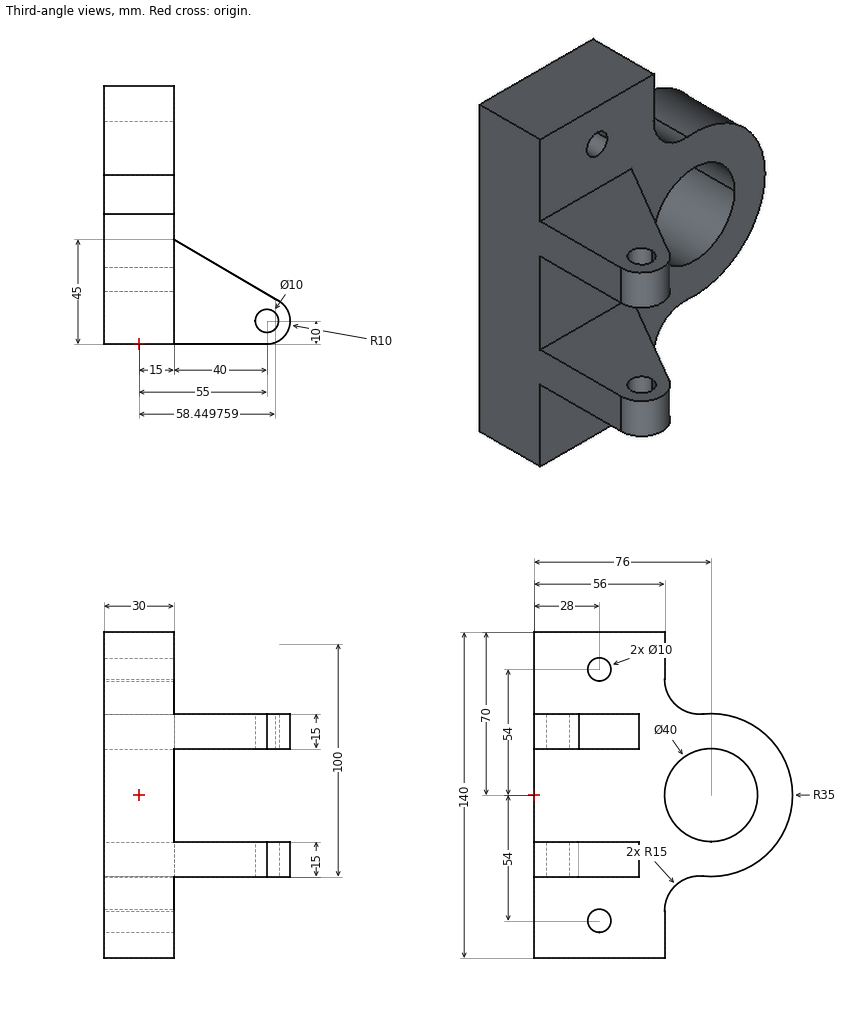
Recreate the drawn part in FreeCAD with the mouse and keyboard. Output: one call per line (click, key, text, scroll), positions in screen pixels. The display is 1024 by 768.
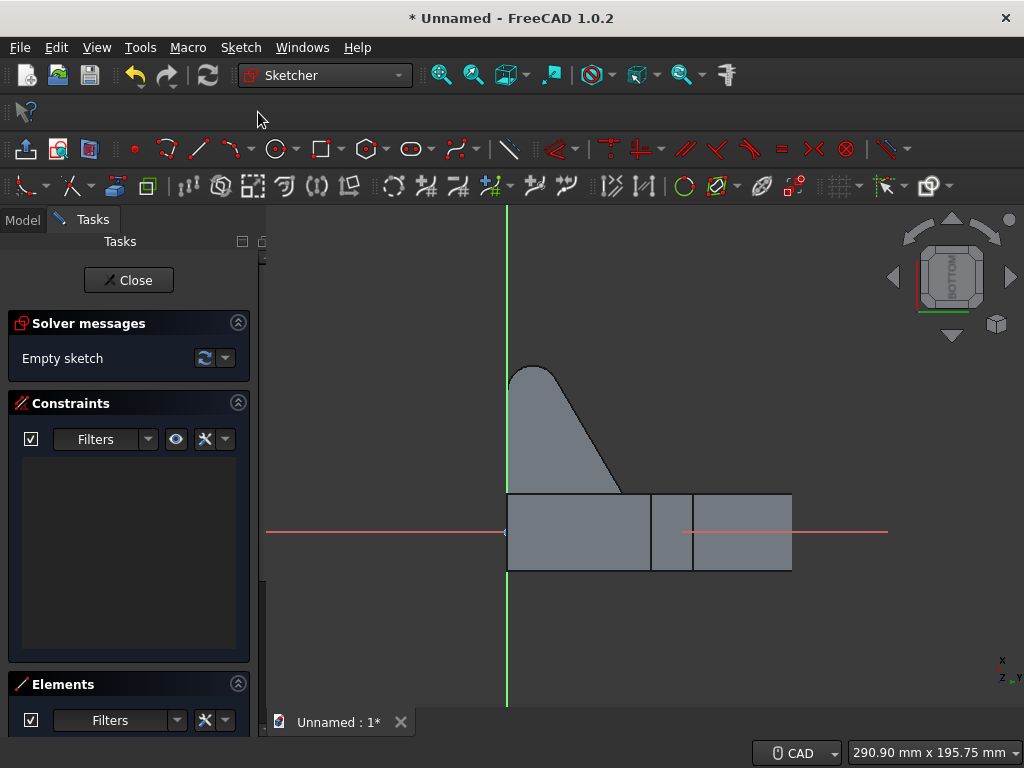
scroll(530, 386, up, 13)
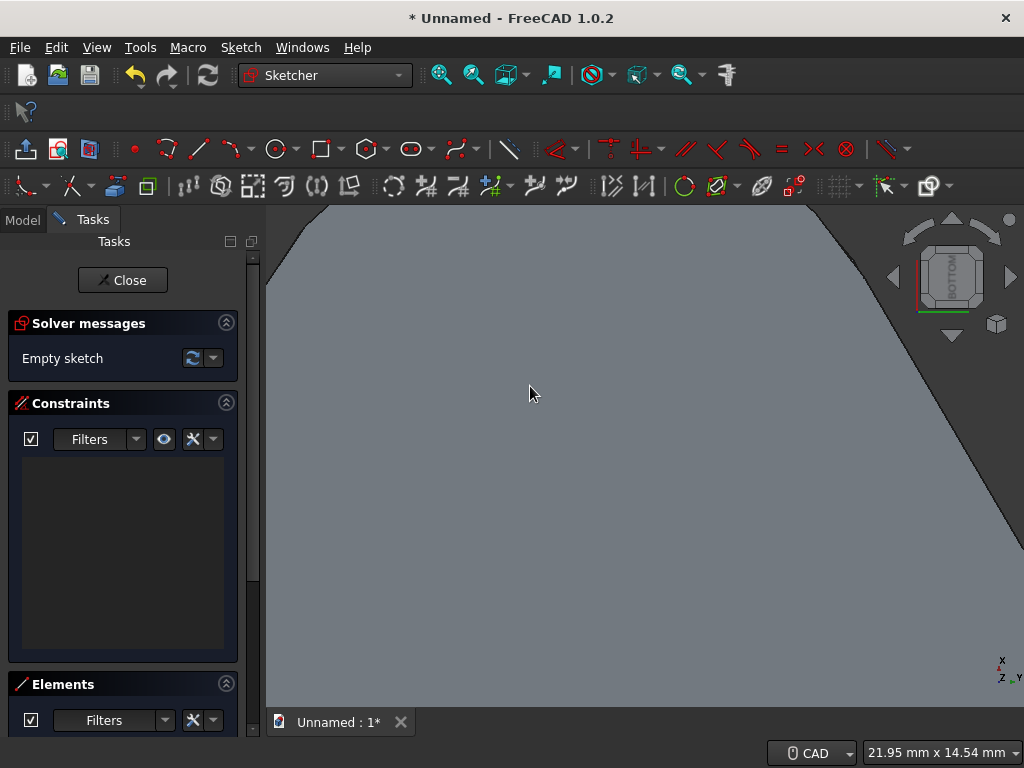
key(g)
key(c)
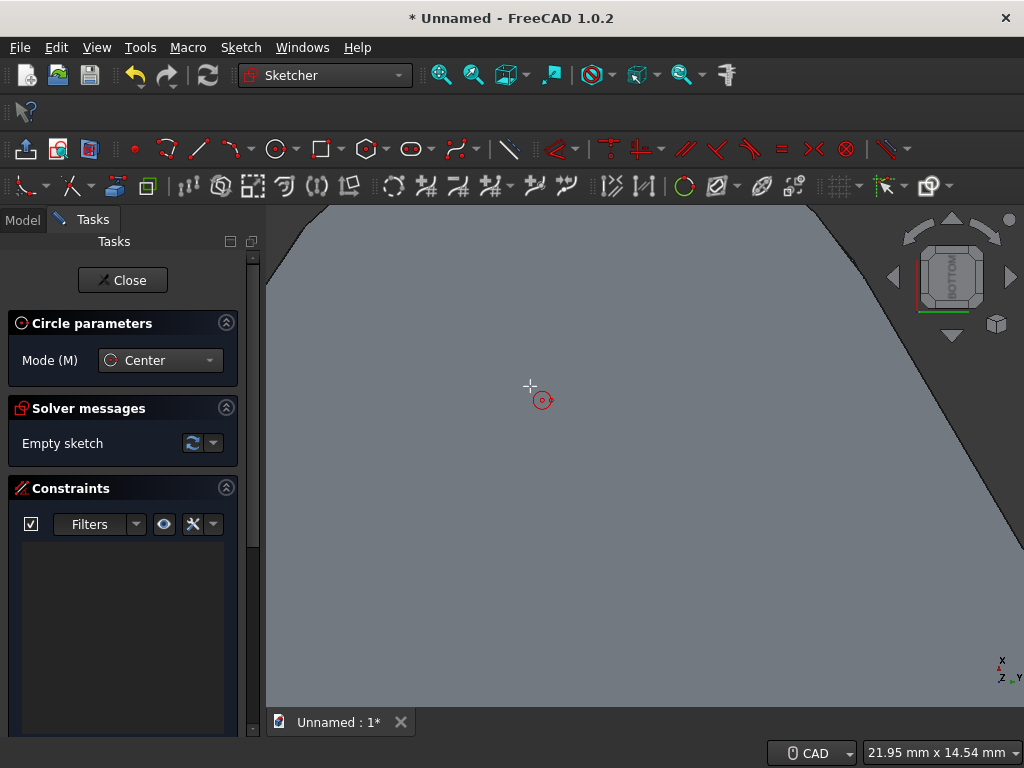
click(567, 452)
click(689, 330)
key(Escape)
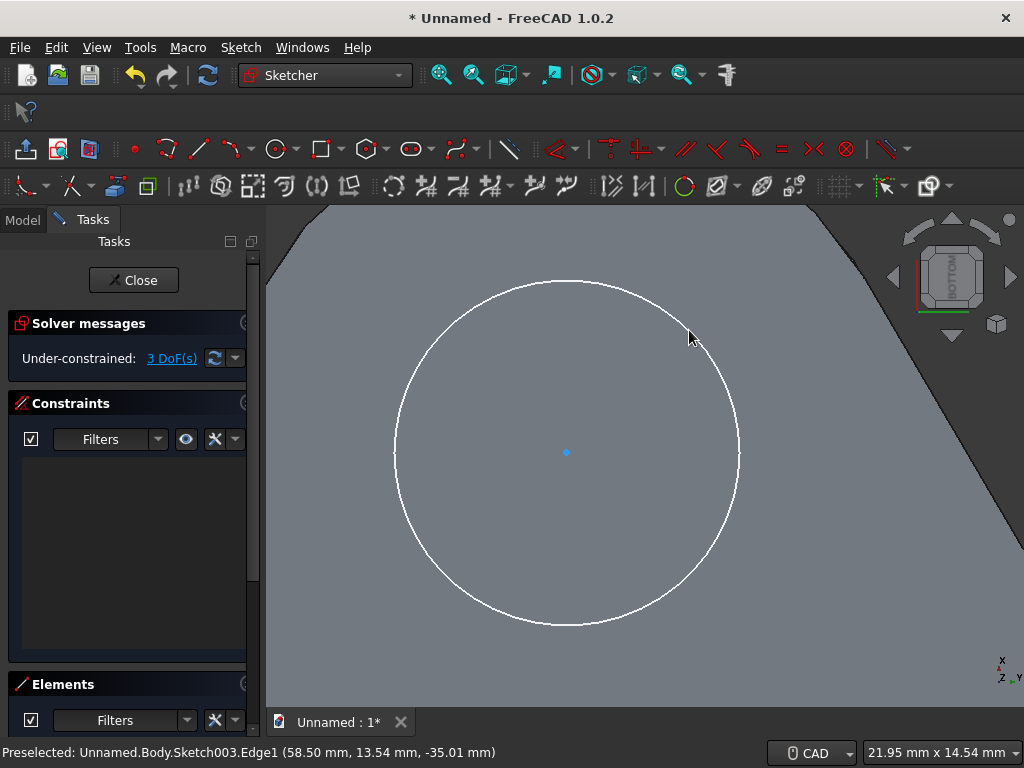
click(556, 150)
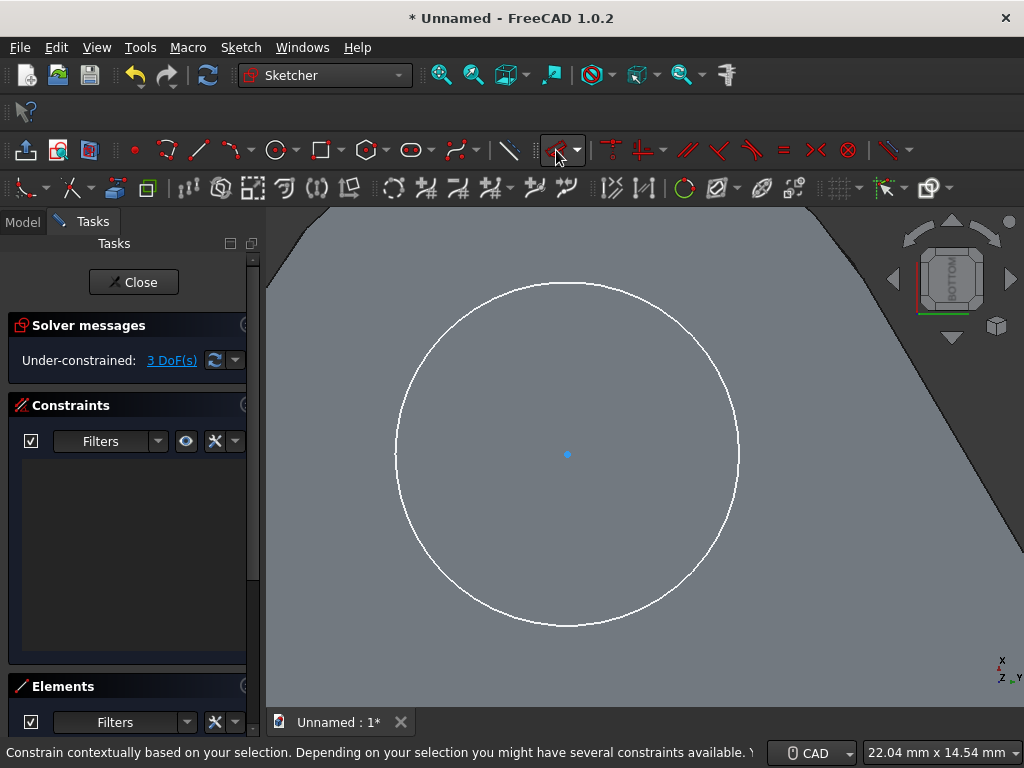
click(688, 332)
click(711, 309)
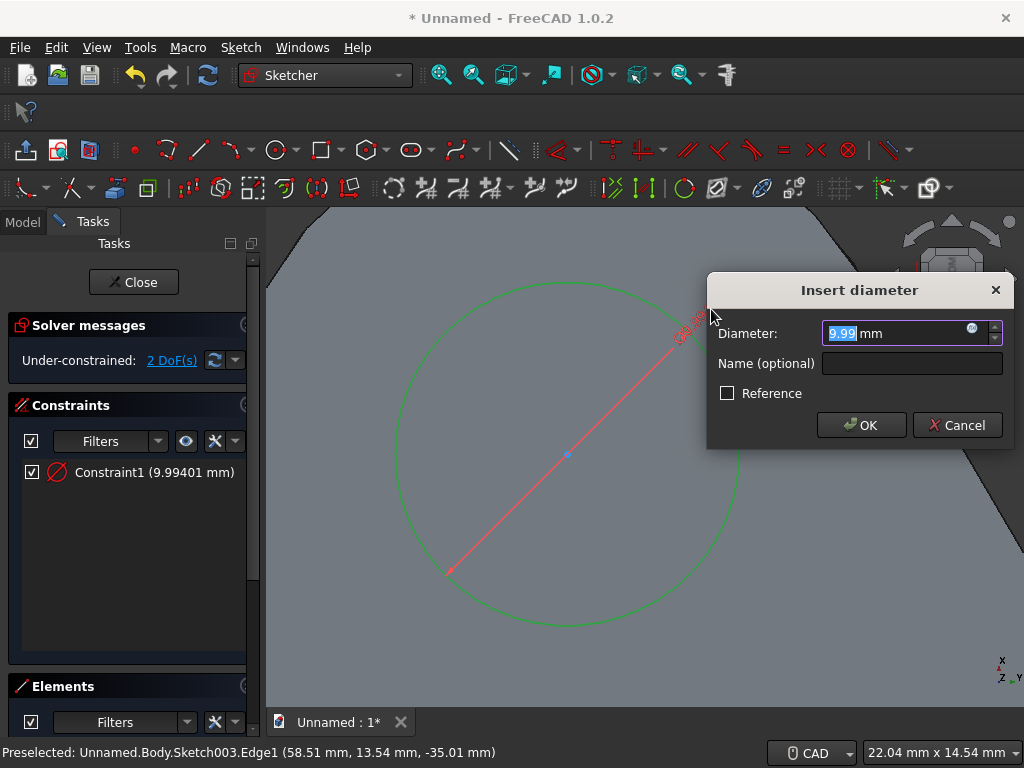
text(10)
key(Return)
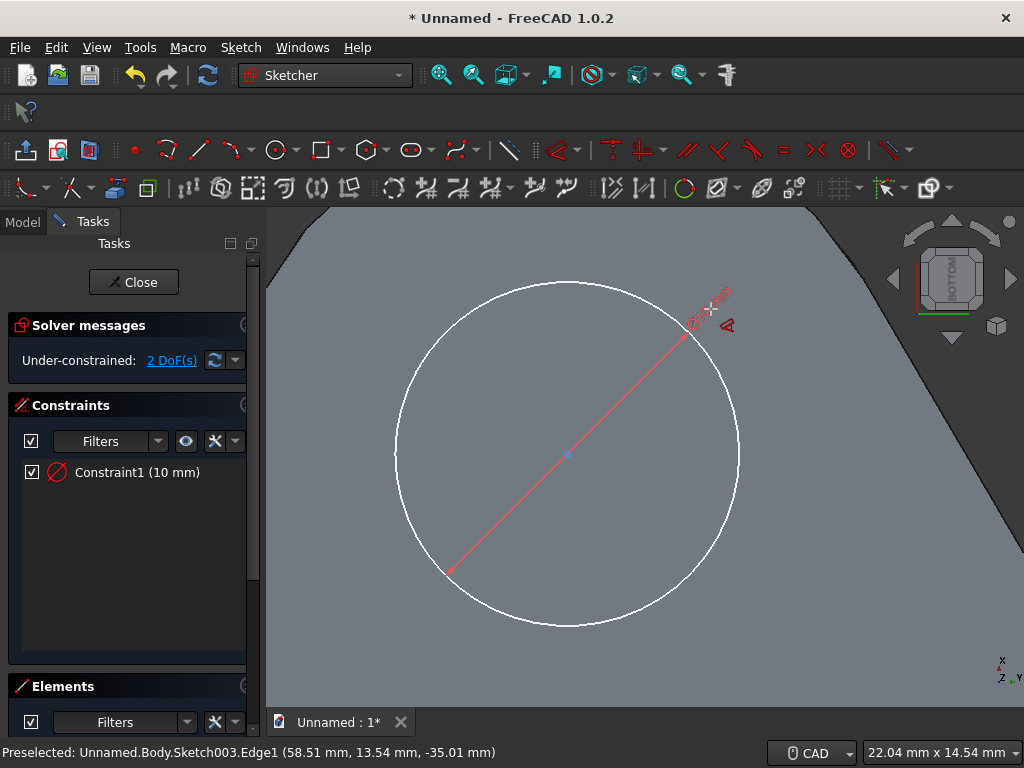
click(567, 454)
click(431, 420)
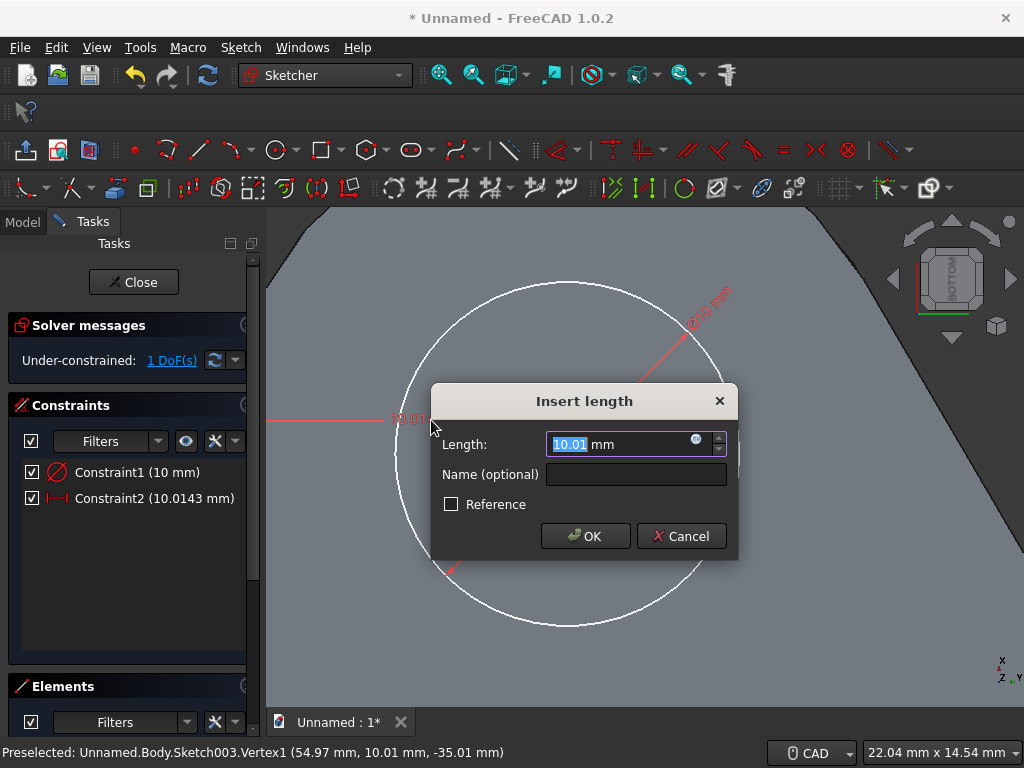
text(10)
key(Return)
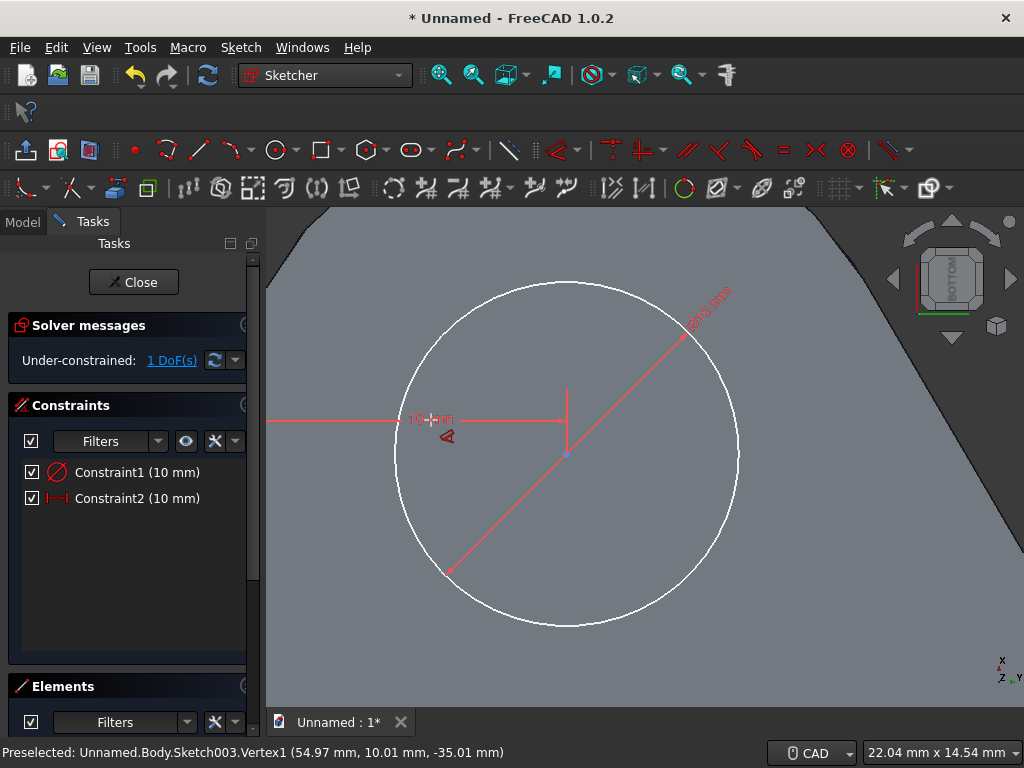
click(567, 454)
click(601, 567)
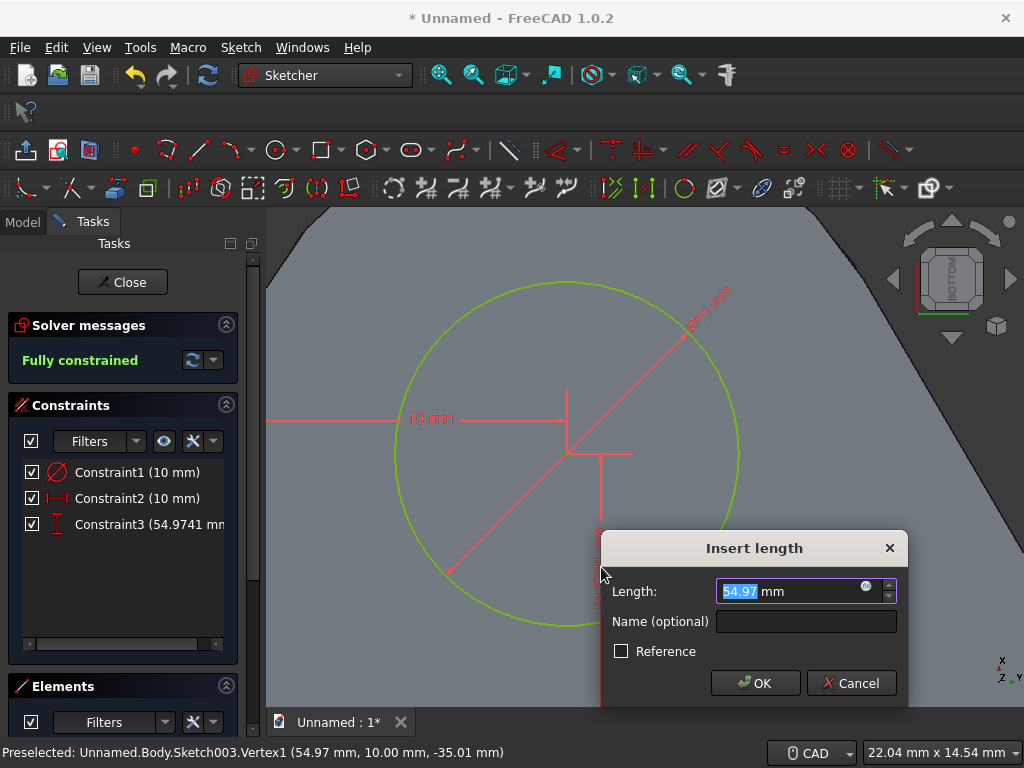
text(55)
key(Return)
key(Escape)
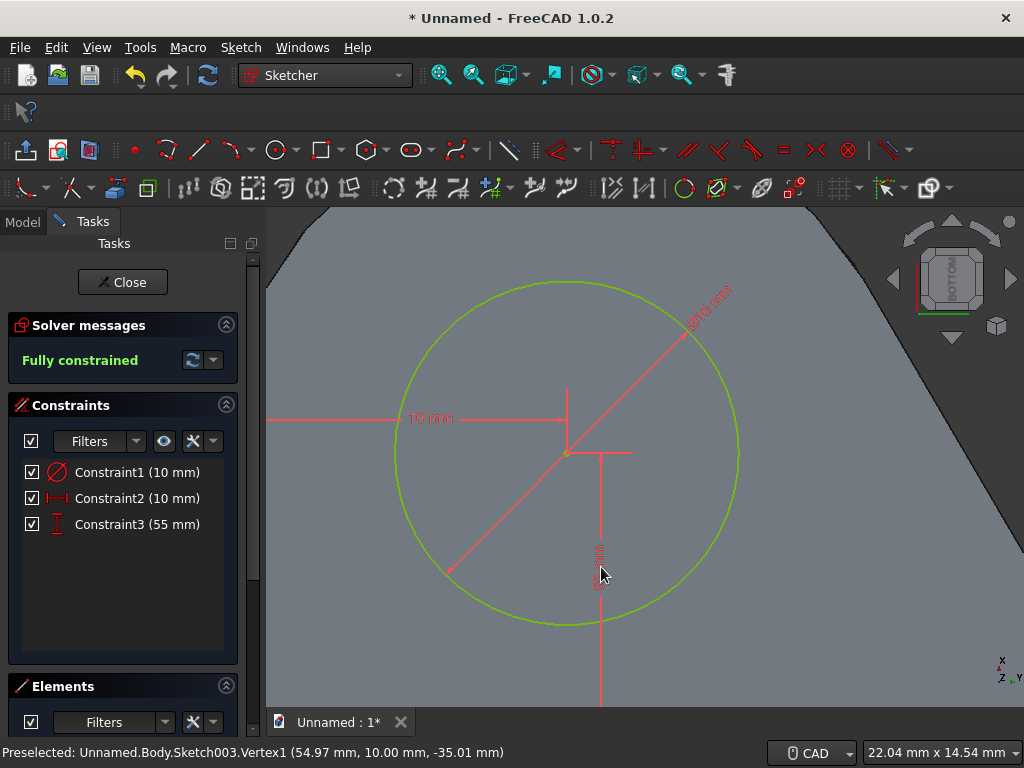
click(123, 282)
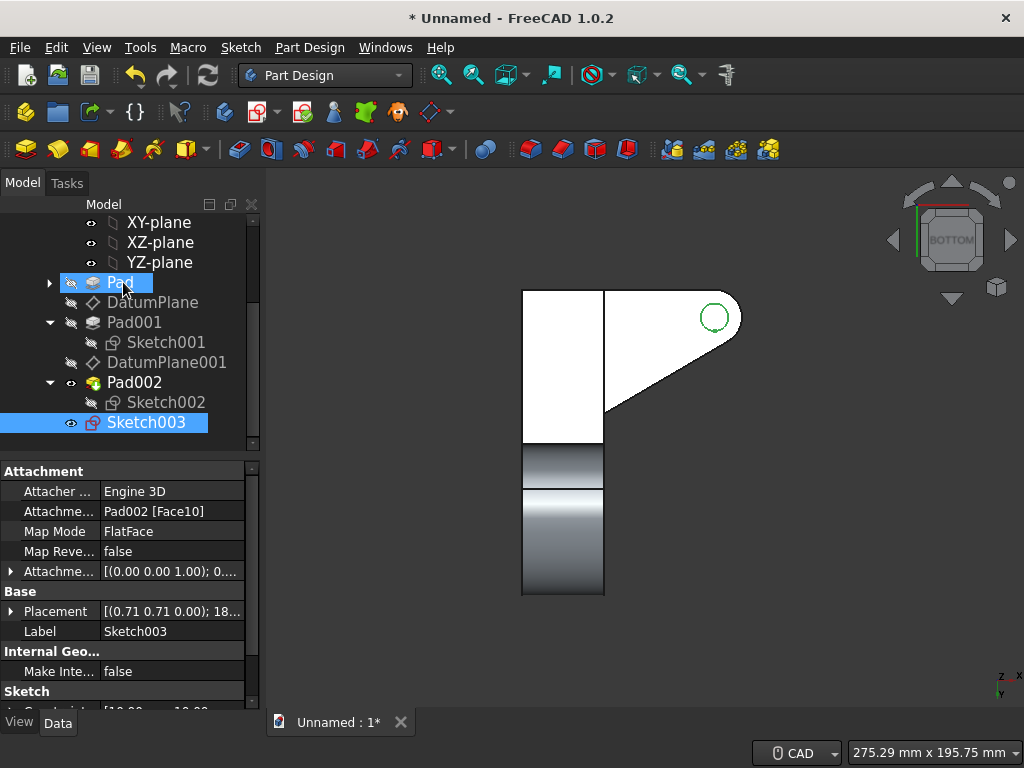
click(240, 150)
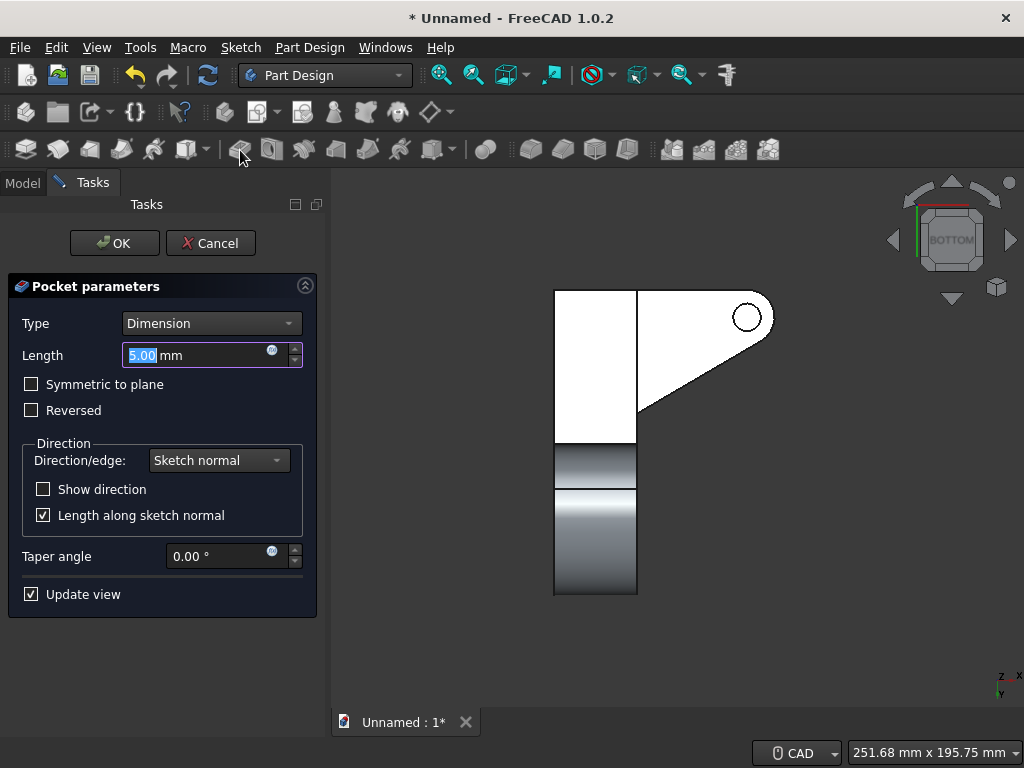
text(100)
key(Tab)